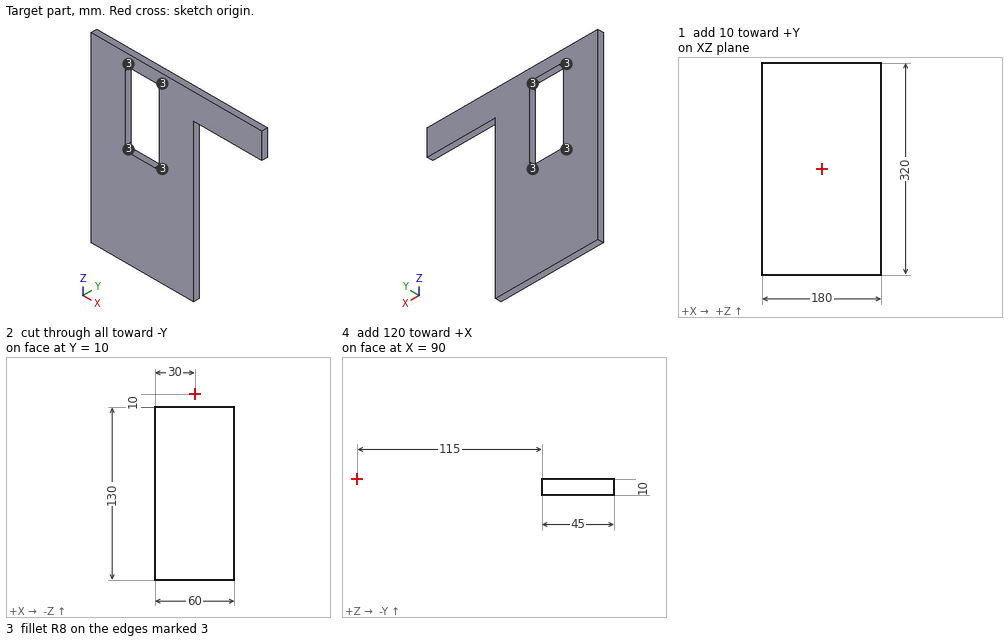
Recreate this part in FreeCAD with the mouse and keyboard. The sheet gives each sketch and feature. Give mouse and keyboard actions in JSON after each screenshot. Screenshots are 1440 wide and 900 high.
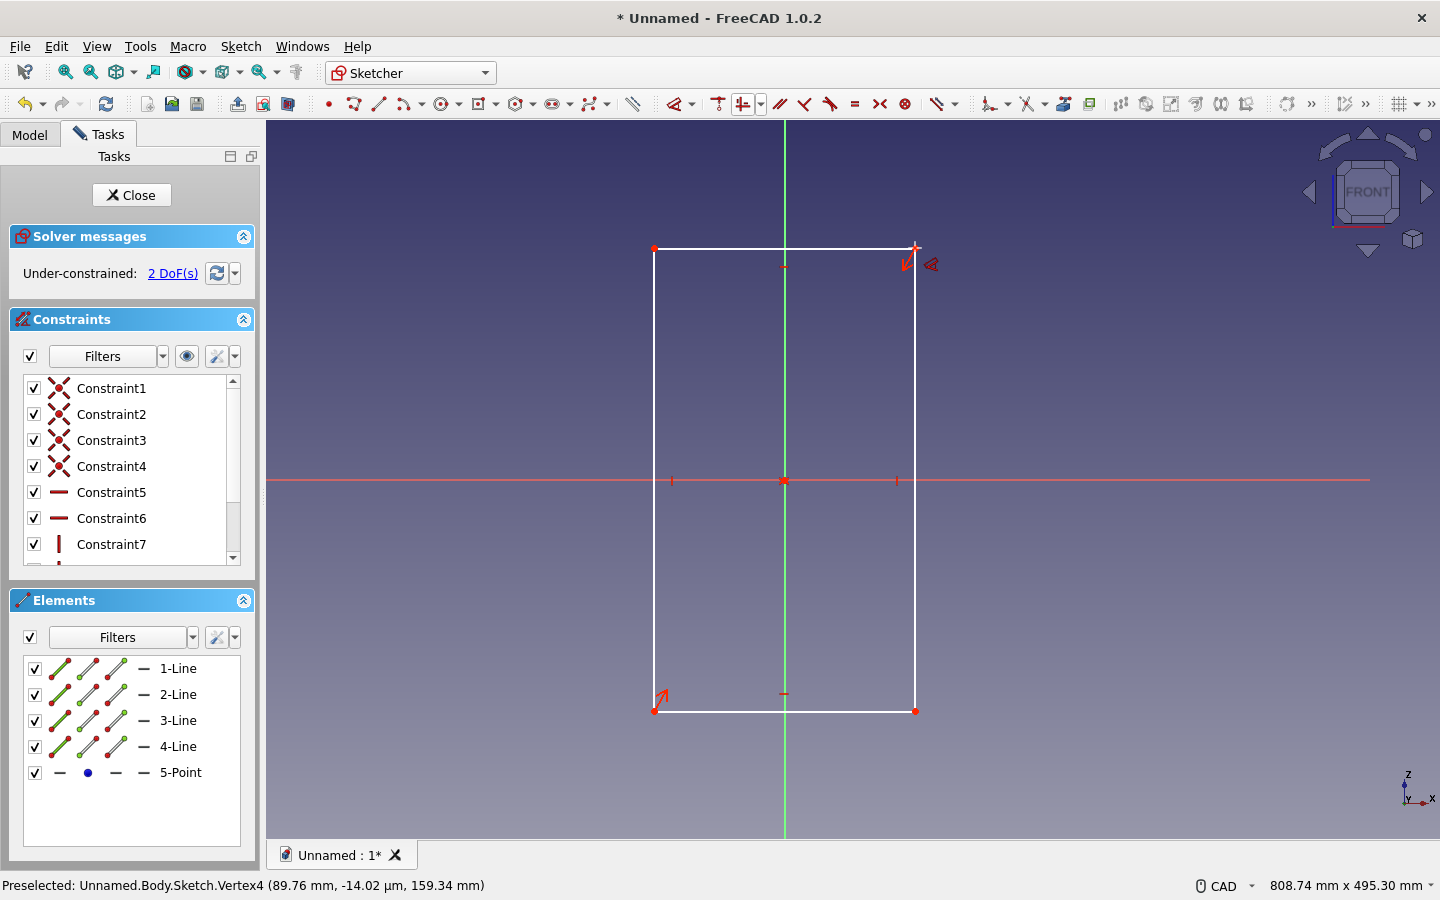
{"action": "left_click", "coordinate": [733, 712]}
{"action": "left_click", "coordinate": [725, 746]}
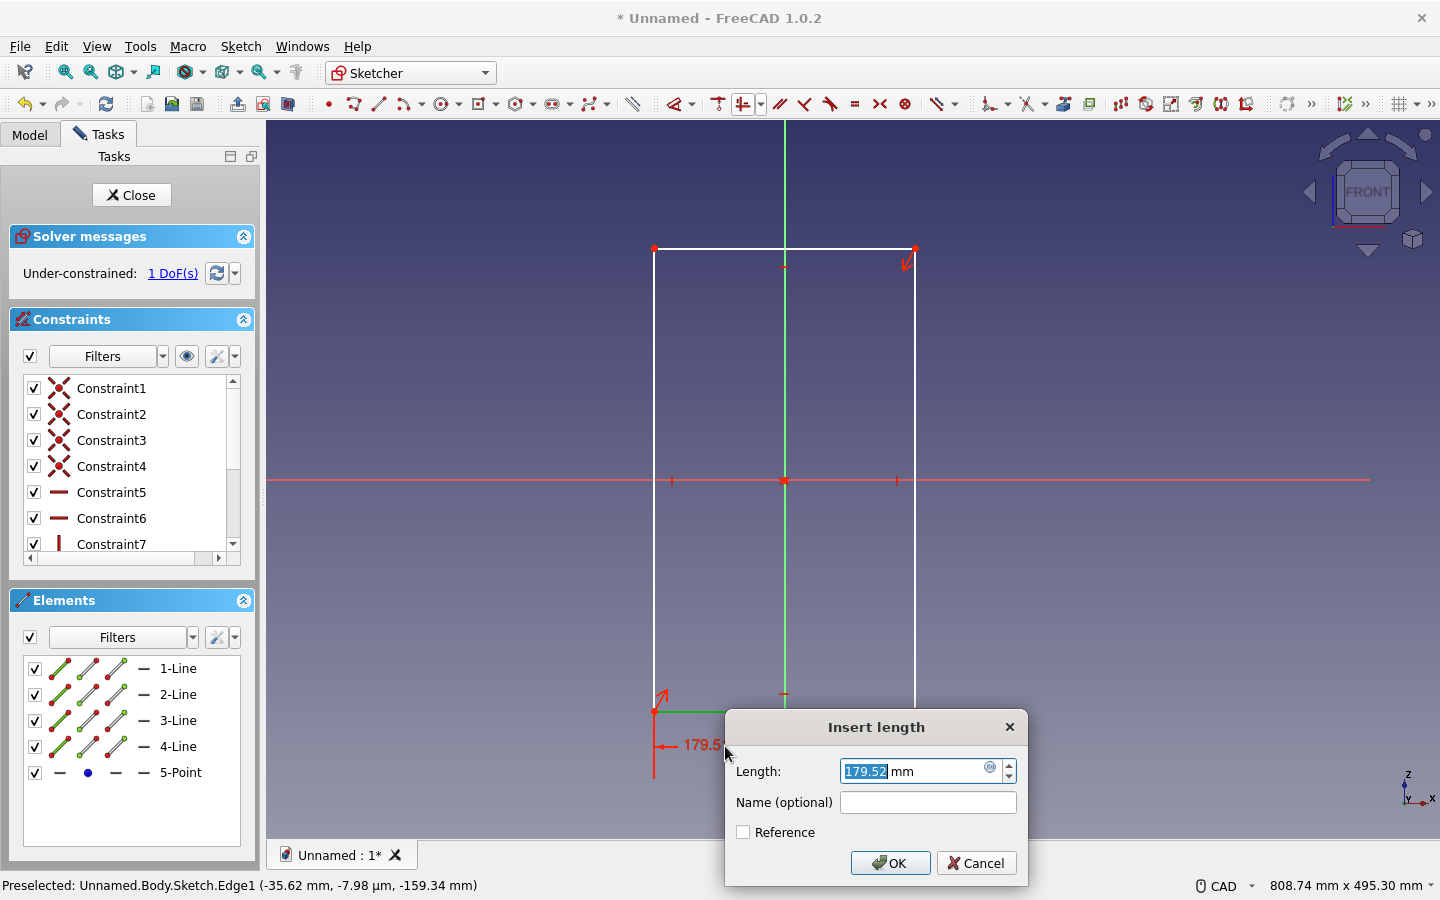
{"action": "type", "text": "180"}
{"action": "key", "text": "Return"}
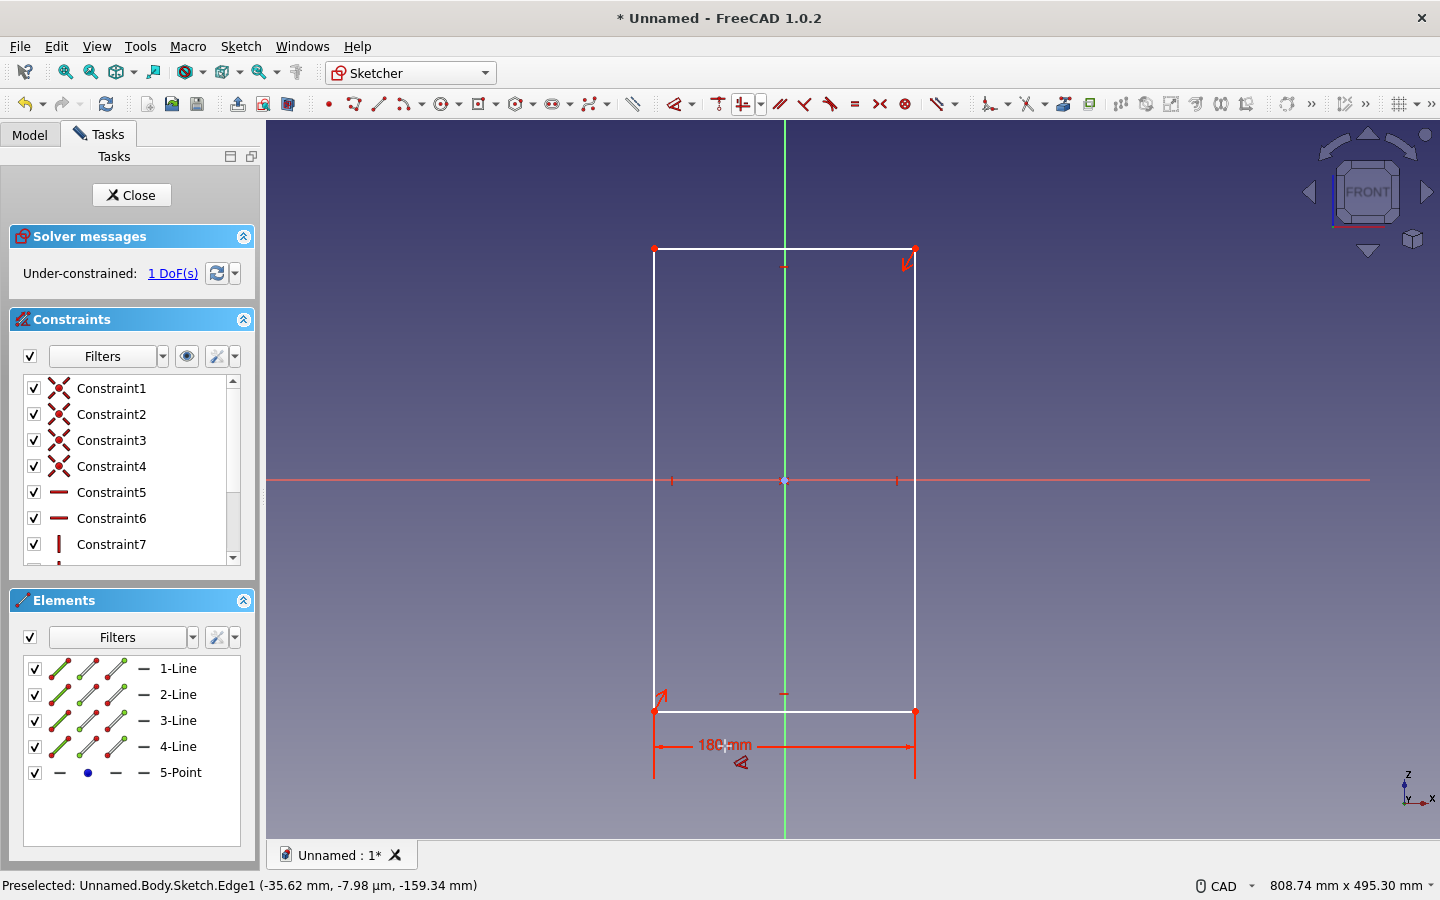
{"action": "left_click", "coordinate": [915, 573]}
{"action": "left_click", "coordinate": [949, 374]}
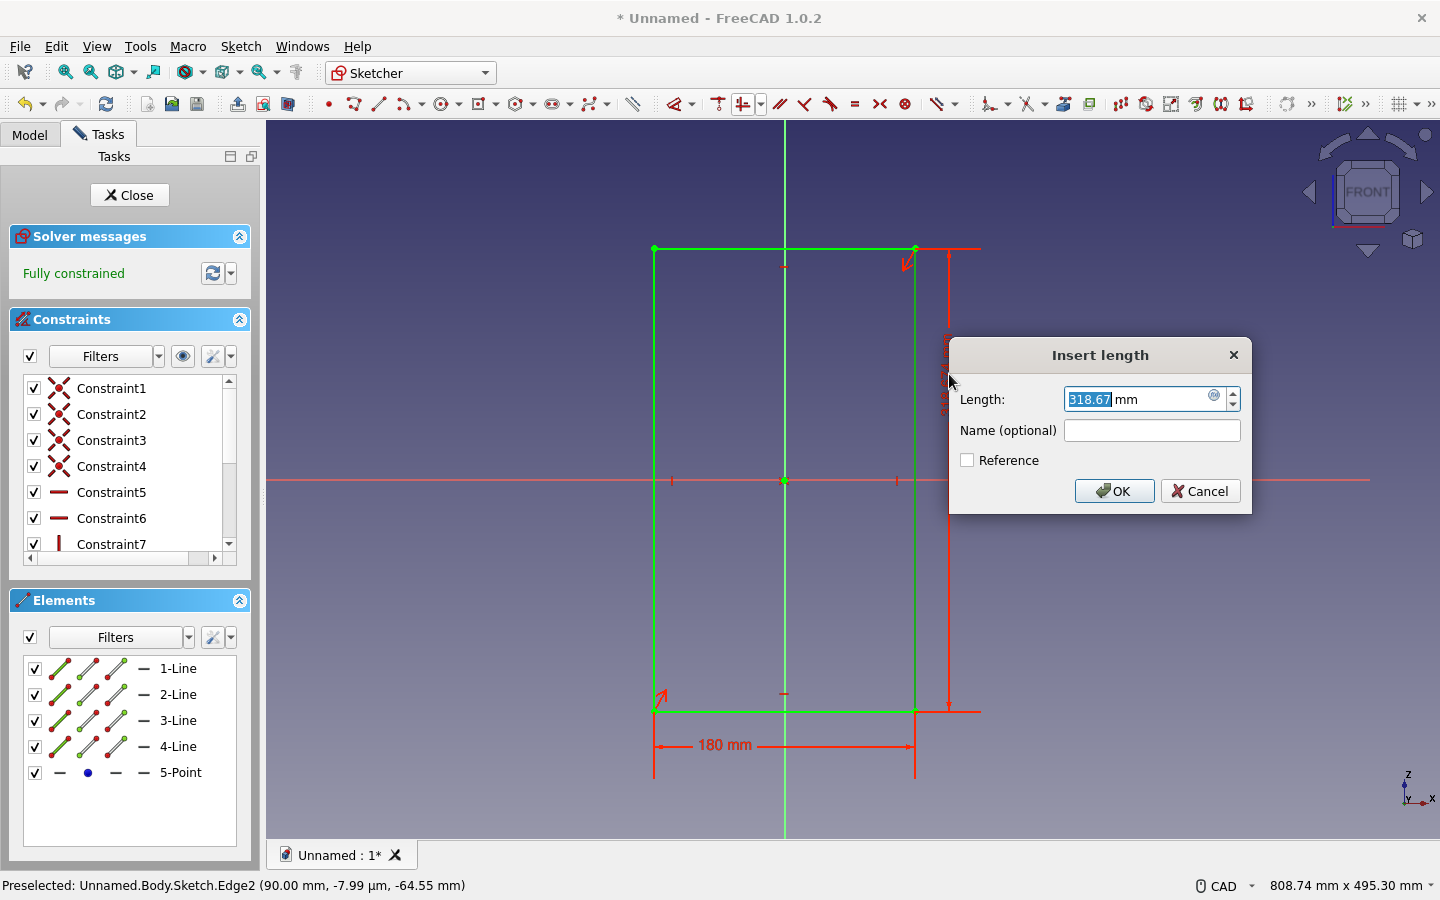
{"action": "type", "text": "320"}
{"action": "key", "text": "Return"}
{"action": "key", "text": "Escape"}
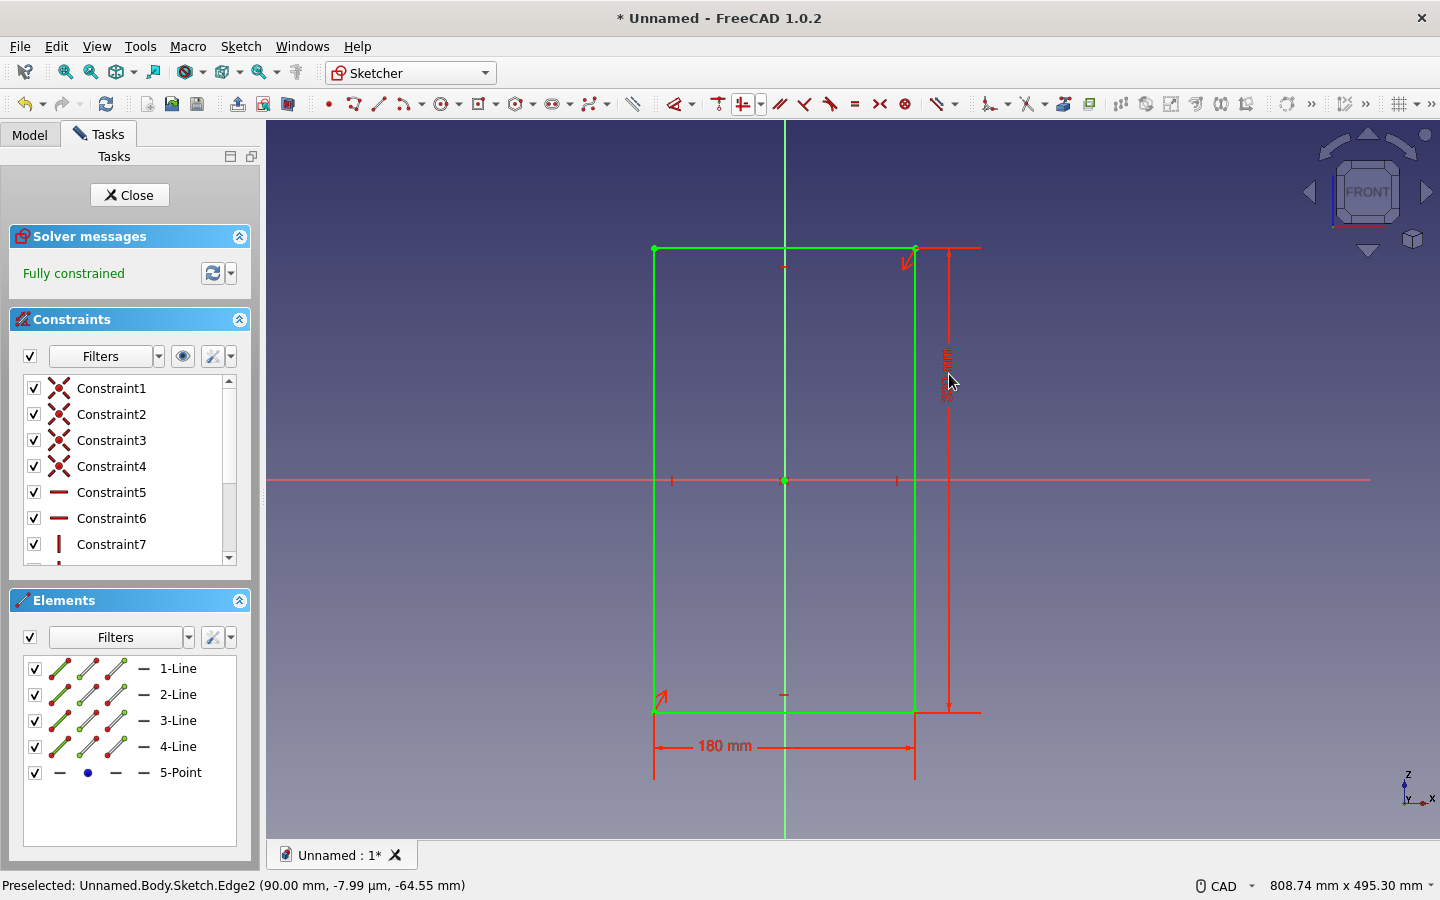
{"action": "left_click", "coordinate": [130, 195]}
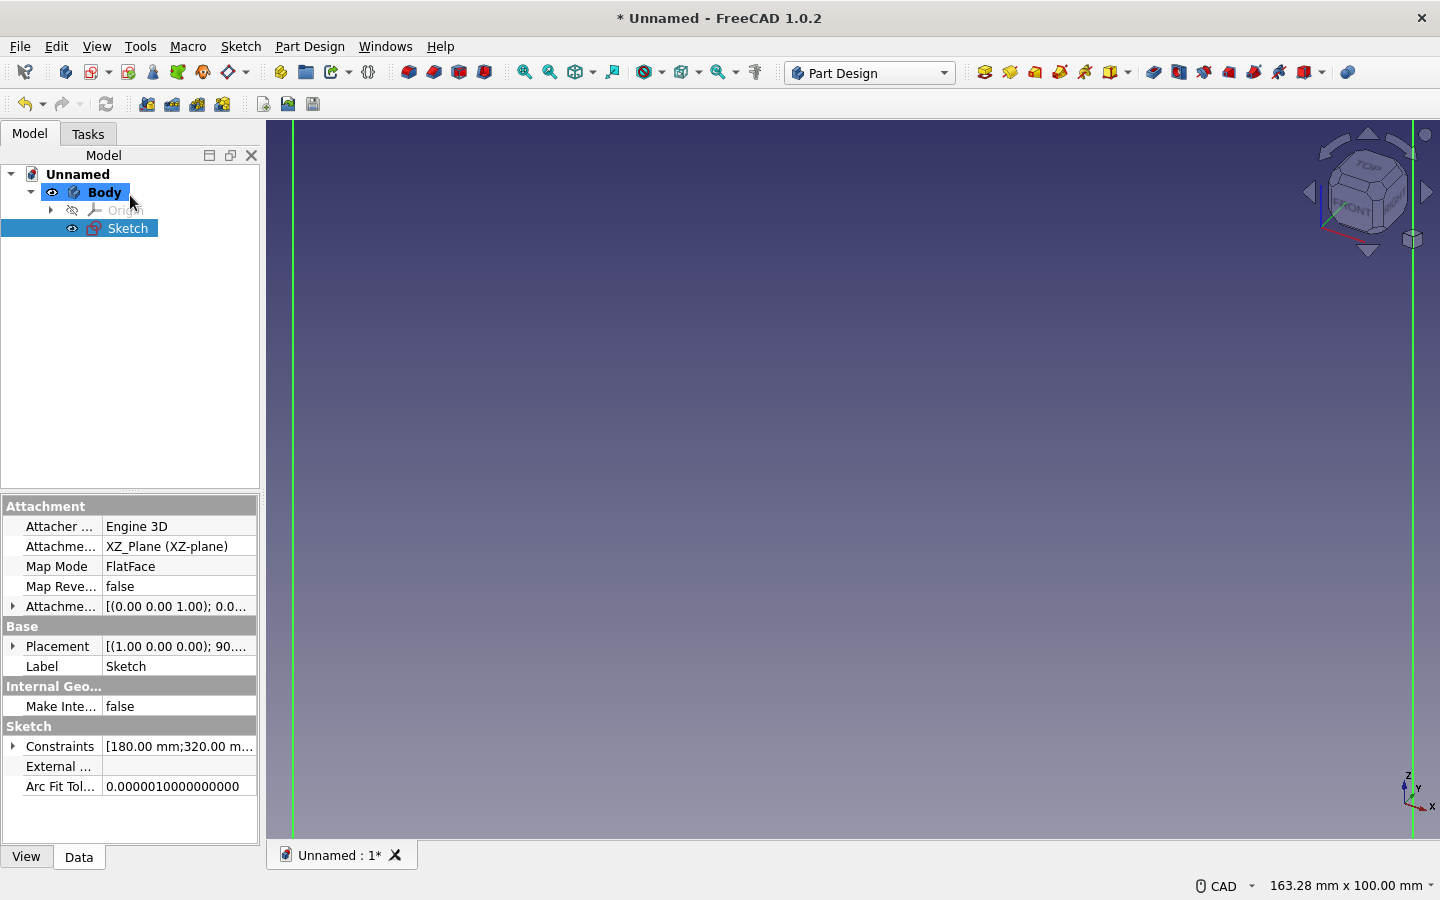
{"action": "left_click", "coordinate": [985, 72]}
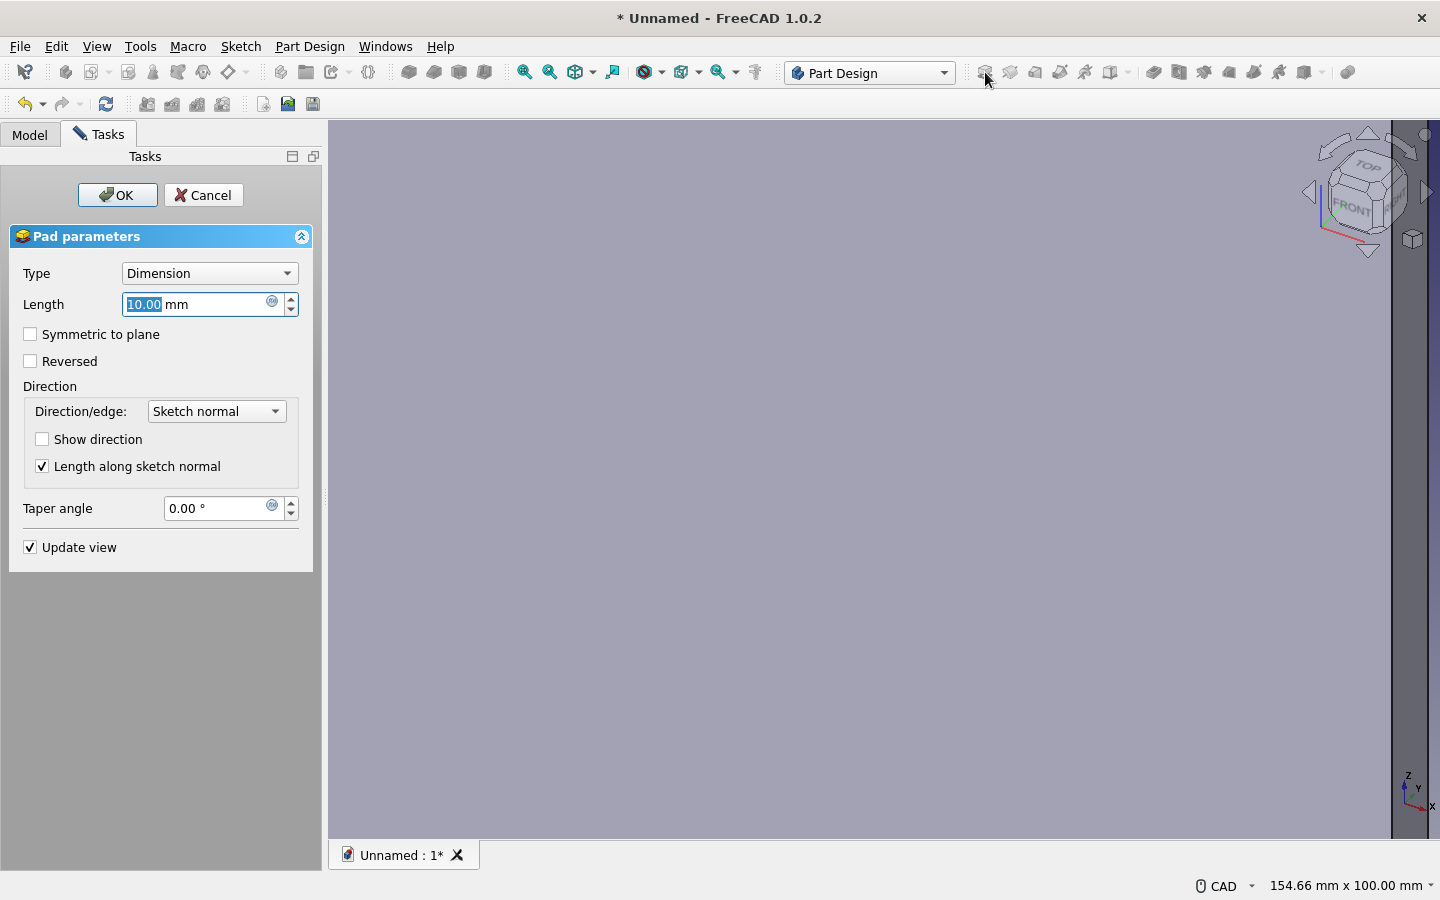
{"action": "type", "text": "10"}
{"action": "key", "text": "Tab"}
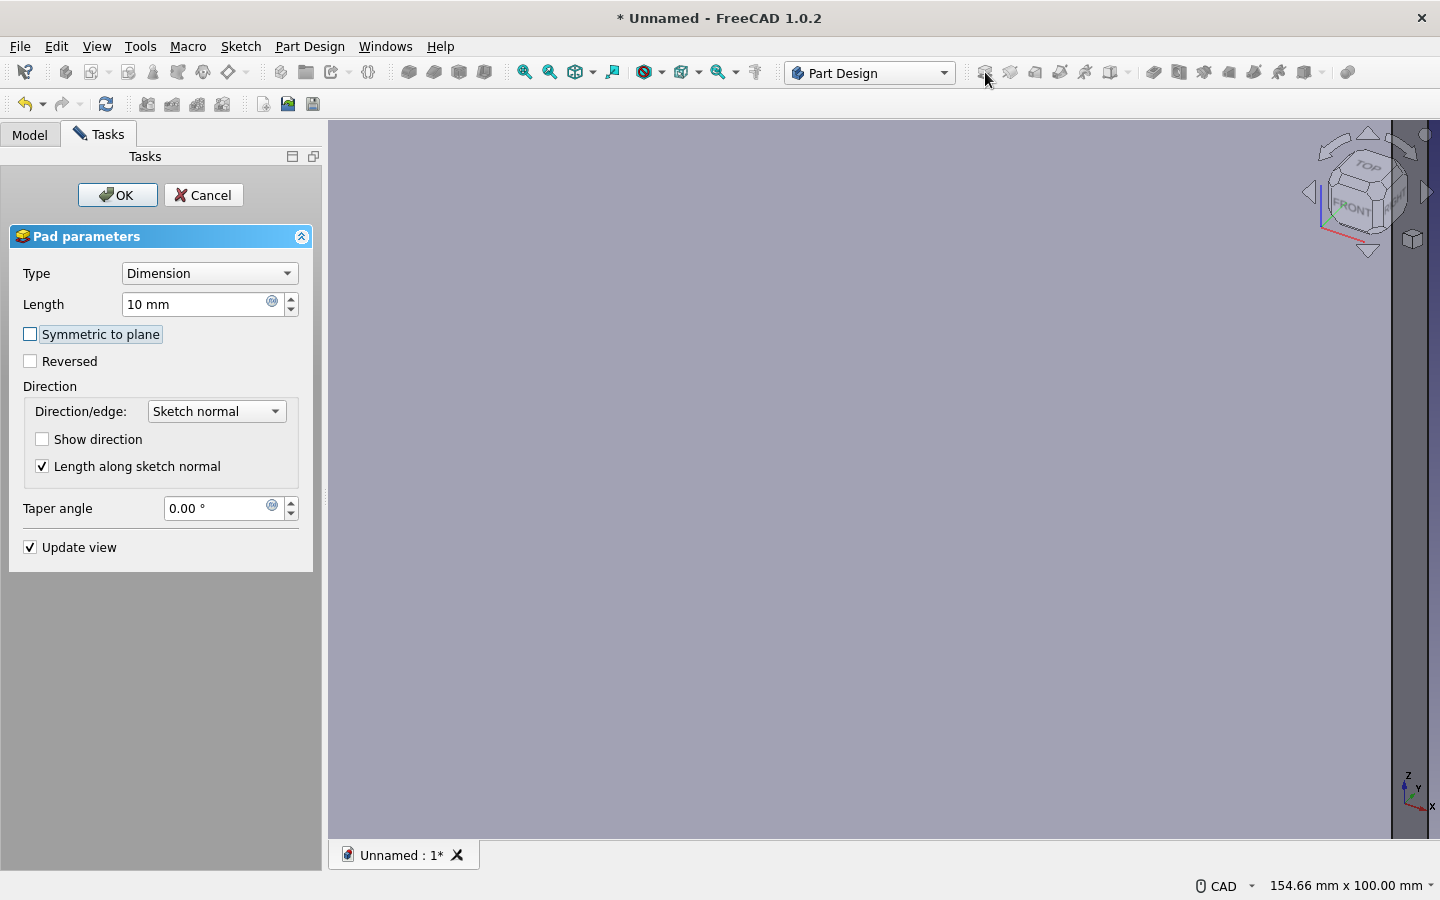
{"action": "left_click", "coordinate": [31, 361]}